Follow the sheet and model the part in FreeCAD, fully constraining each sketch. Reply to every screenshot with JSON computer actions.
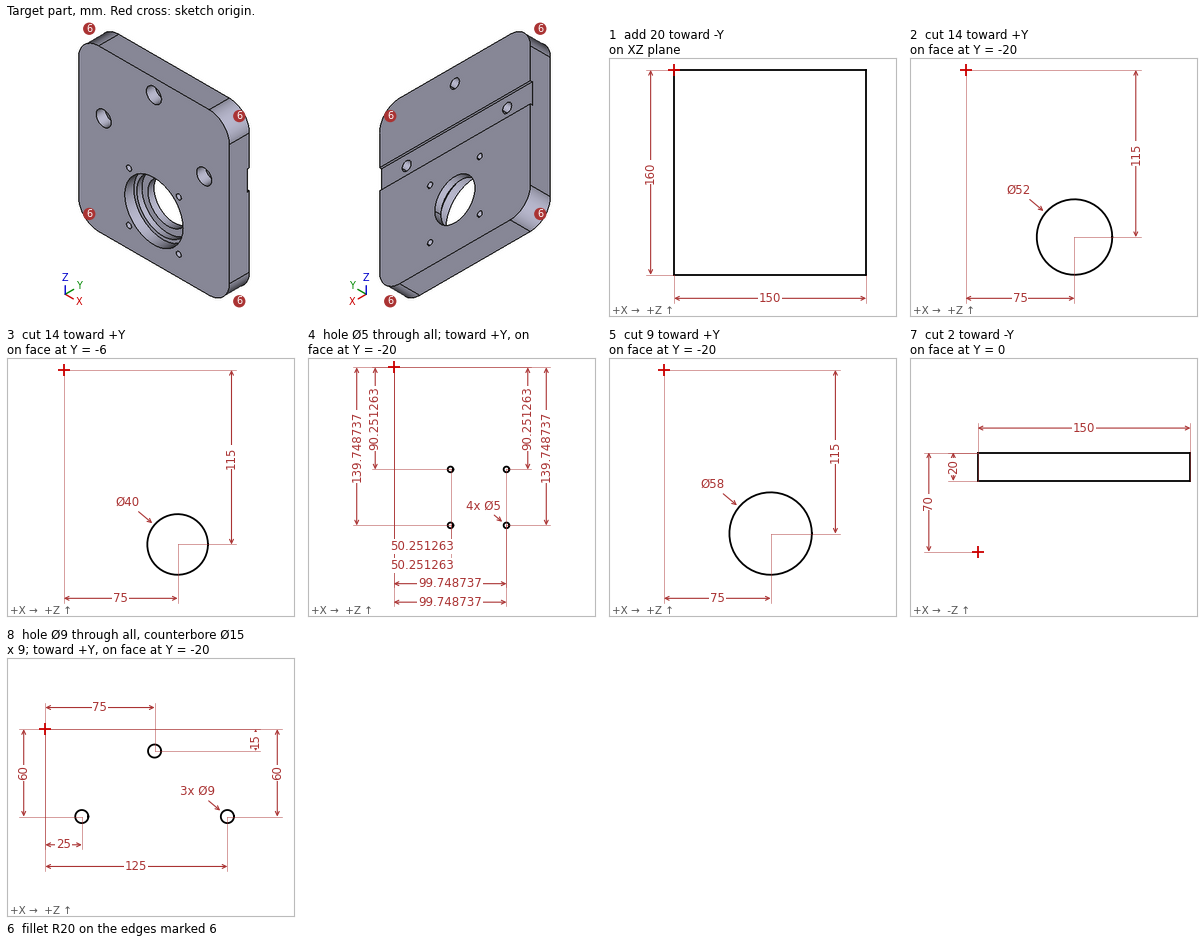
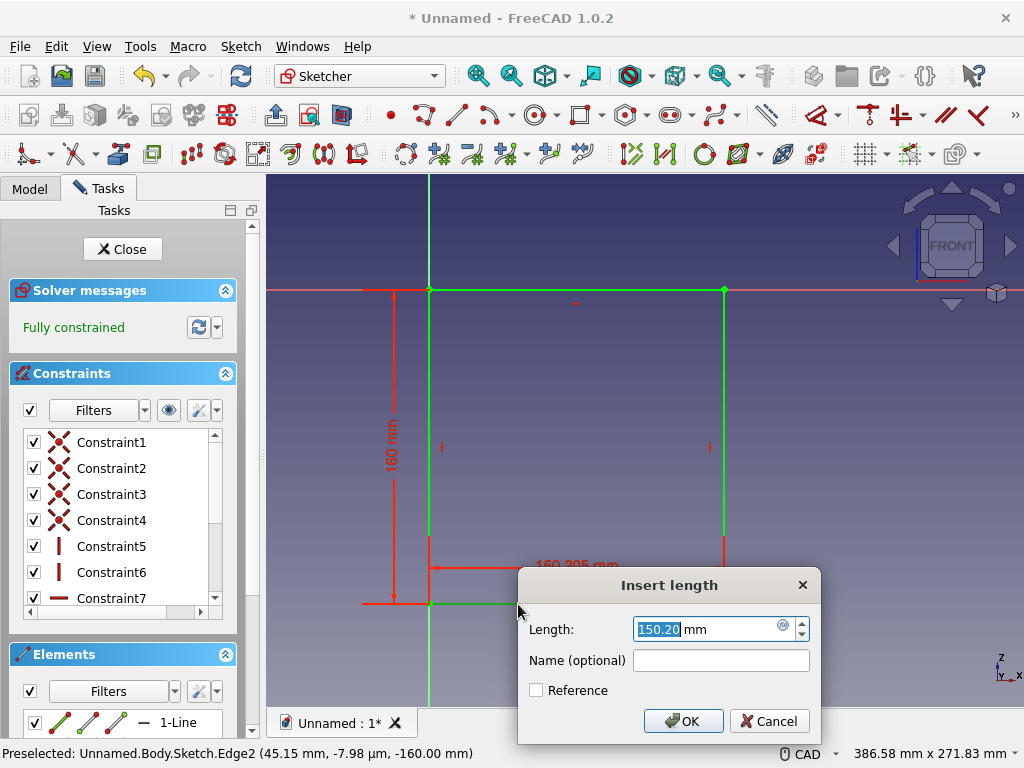
{"action": "type", "text": "150"}
{"action": "key", "text": "Return"}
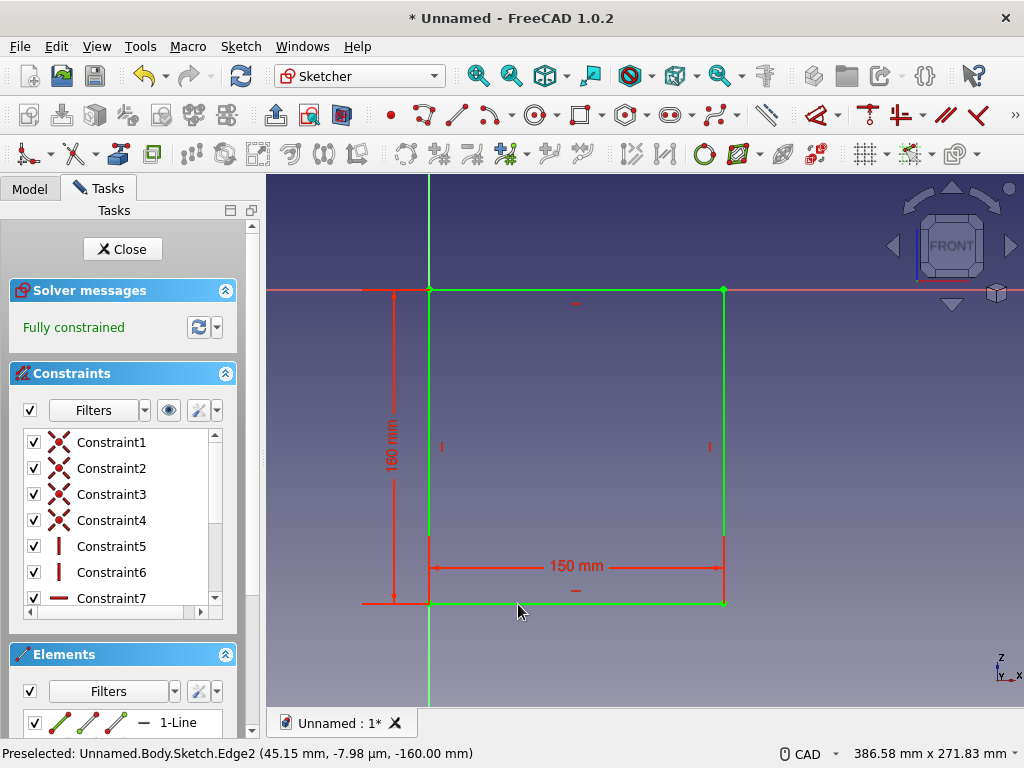
{"action": "left_click", "coordinate": [123, 249]}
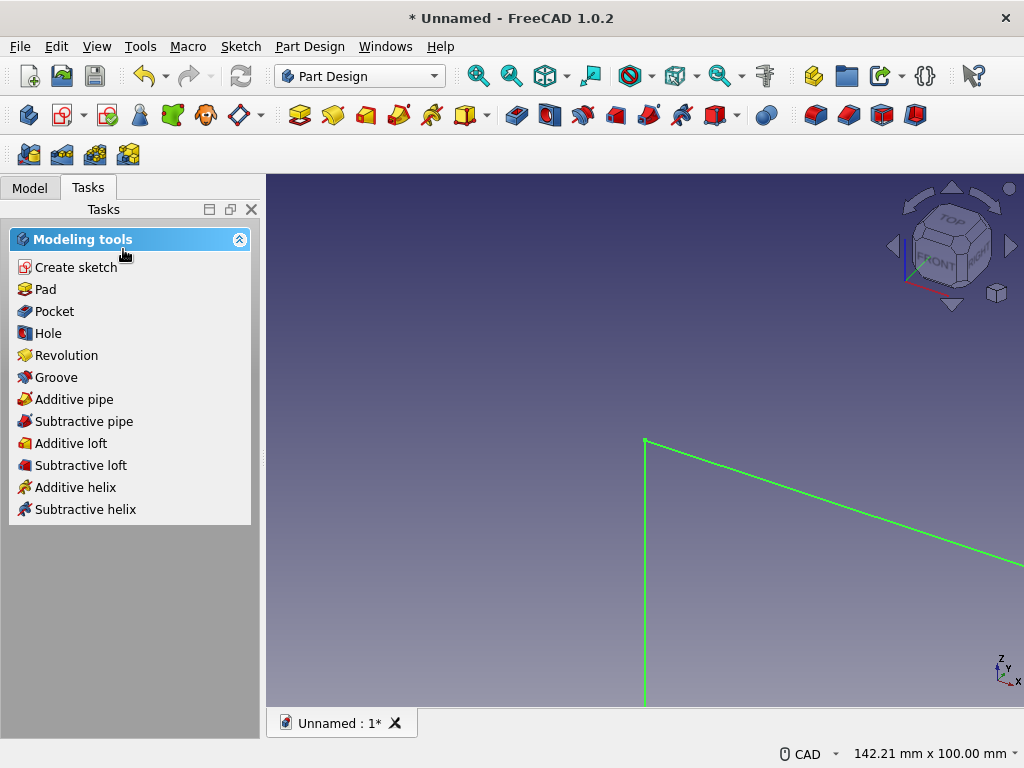
{"action": "left_click", "coordinate": [300, 116]}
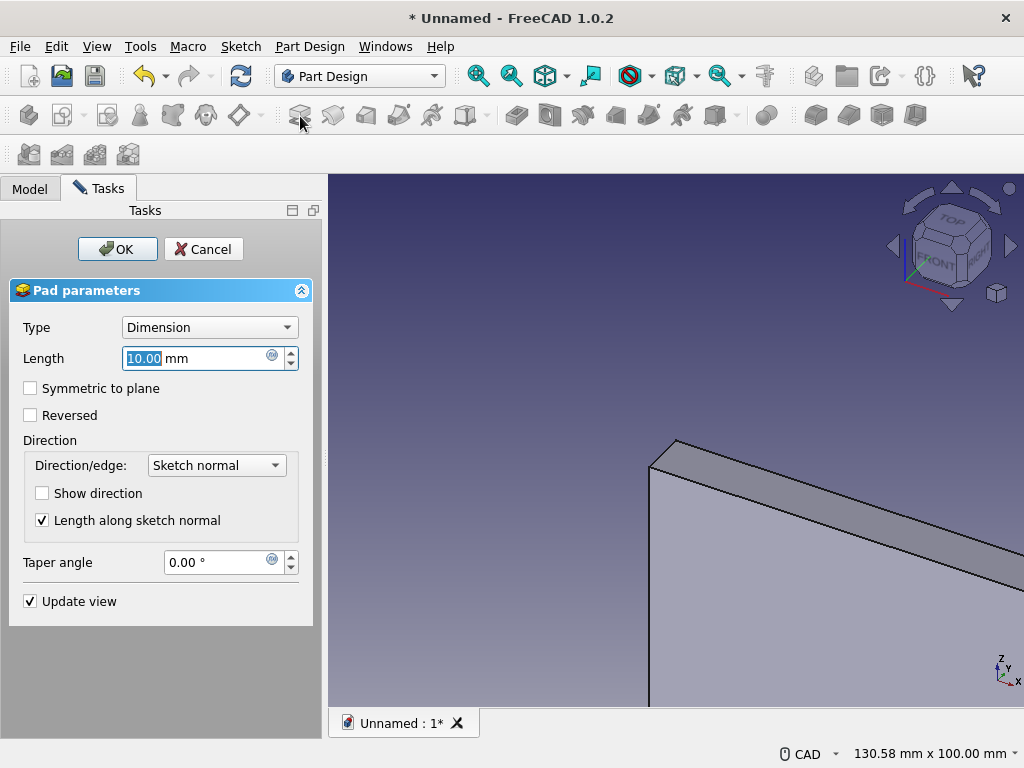
{"action": "type", "text": "20"}
{"action": "key", "text": "Tab"}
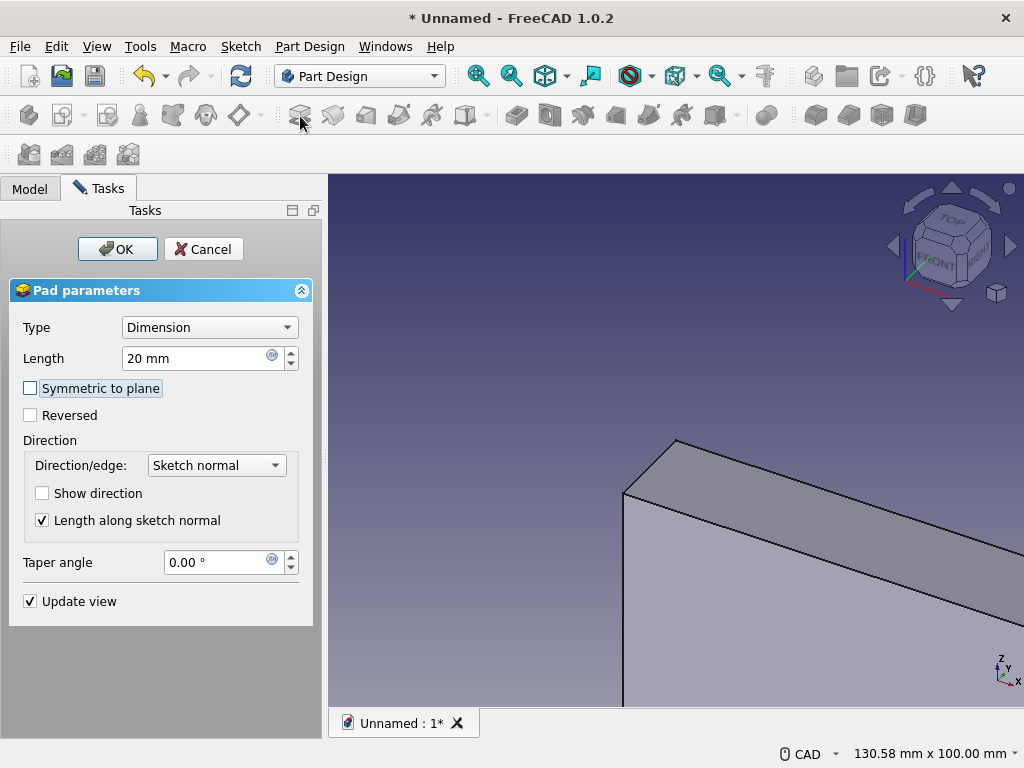
{"action": "left_click", "coordinate": [118, 249]}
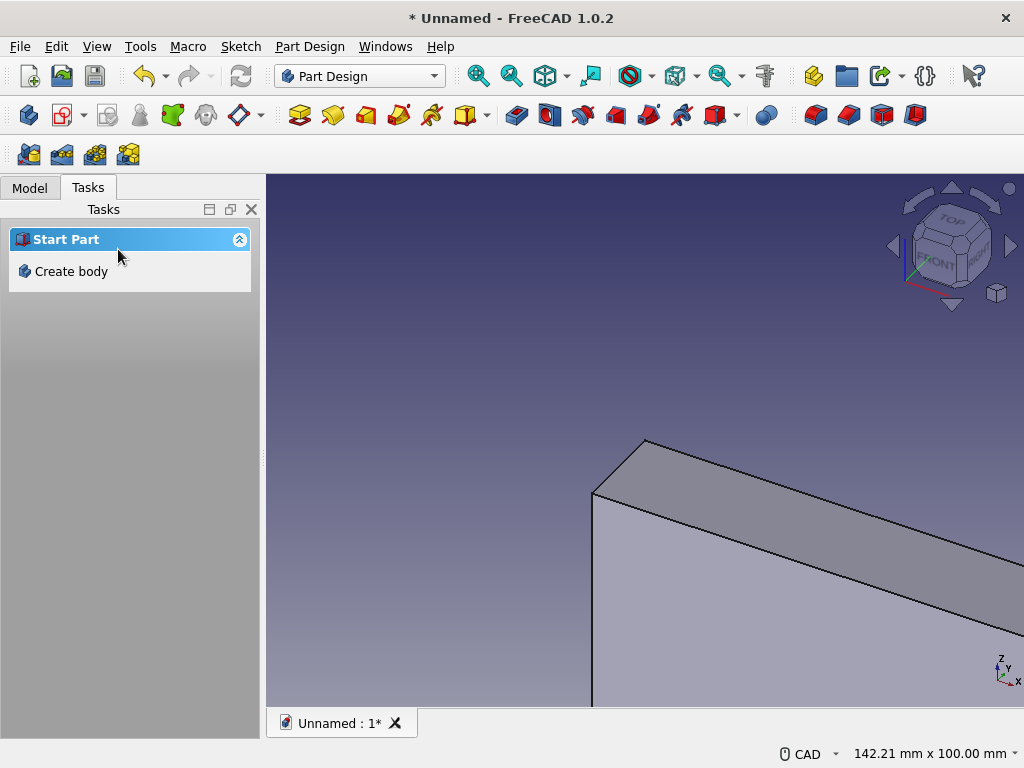
{"action": "left_click", "coordinate": [479, 76]}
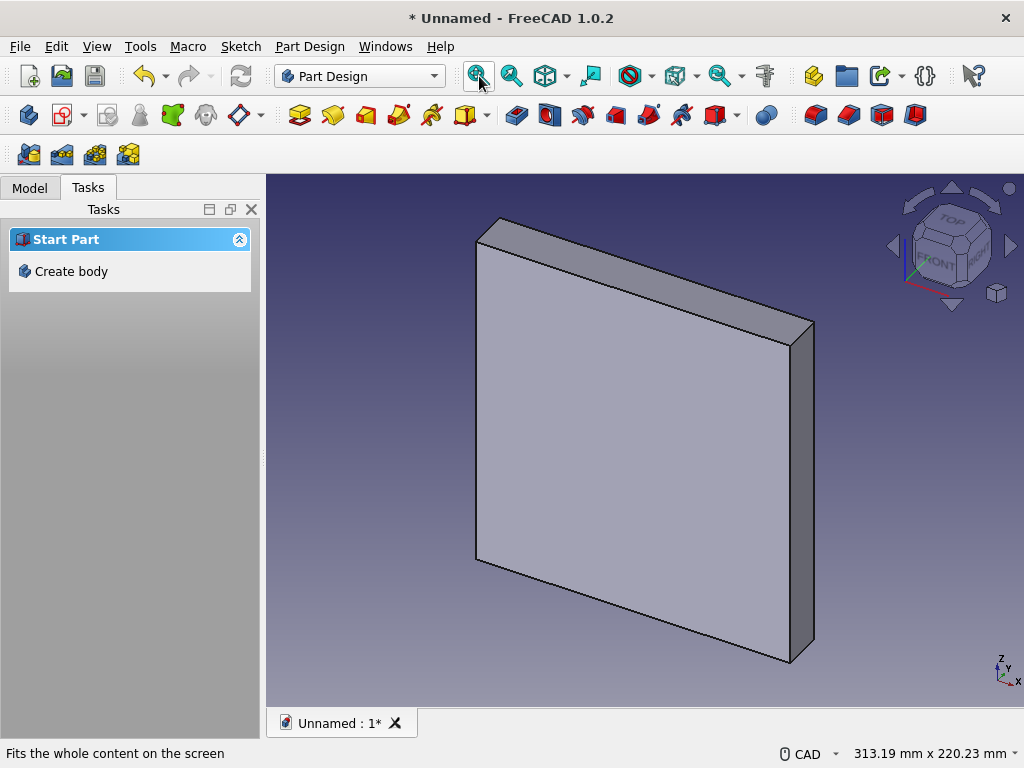
{"action": "left_click", "coordinate": [633, 452]}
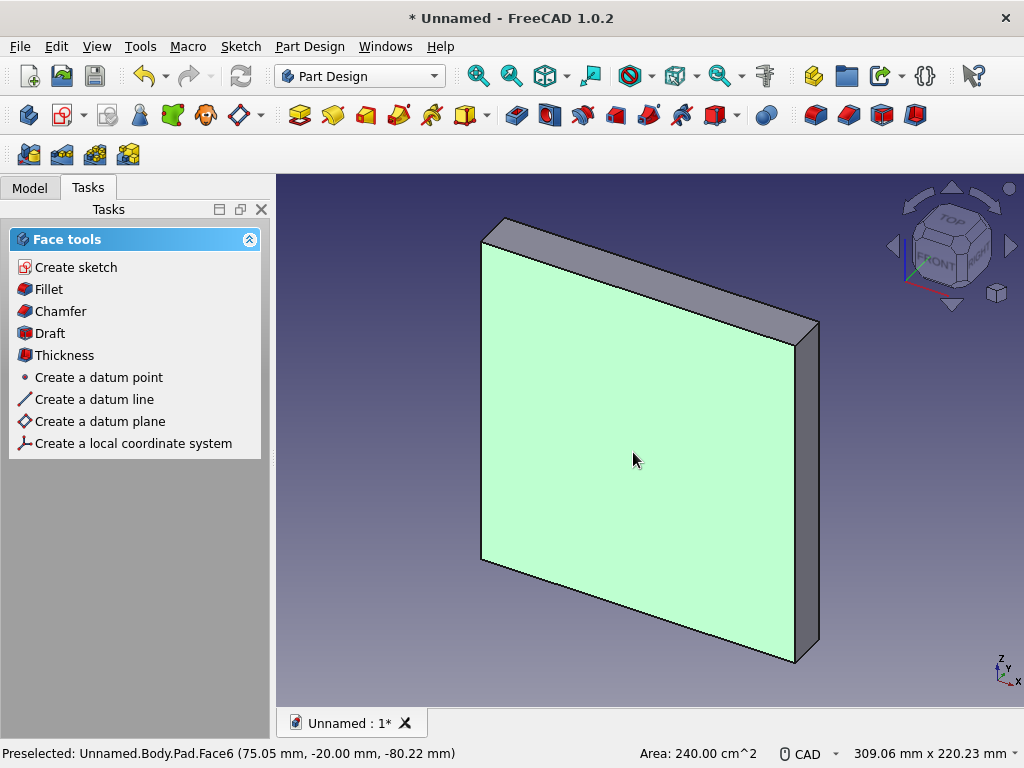
{"action": "left_click", "coordinate": [62, 116]}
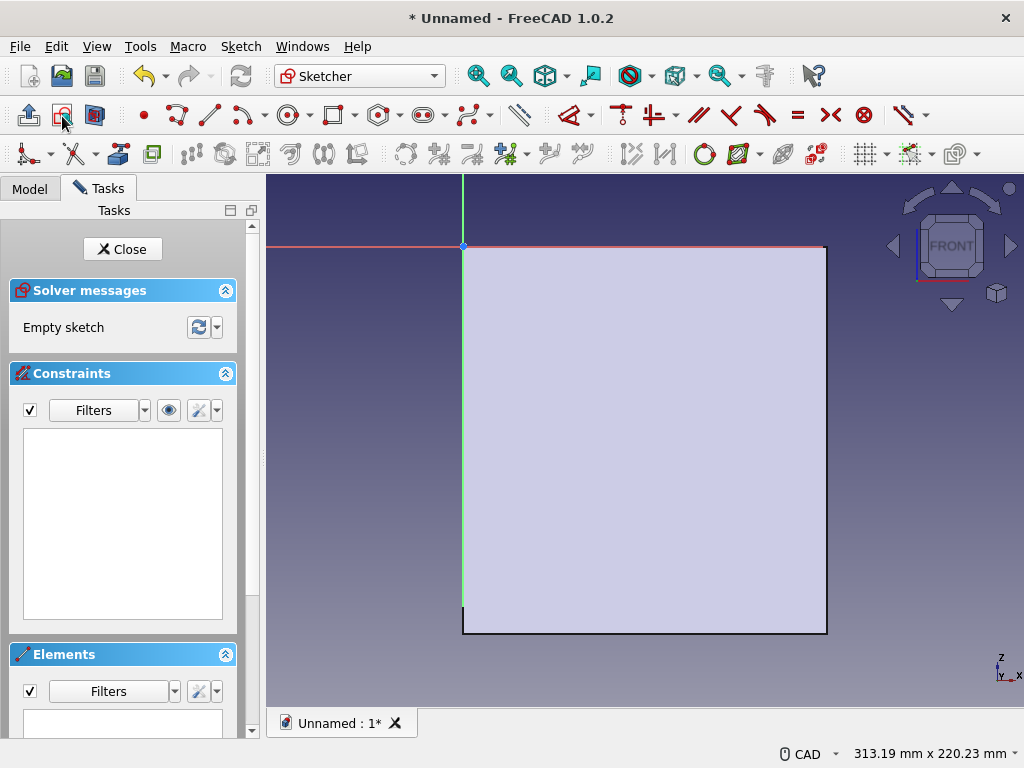
{"action": "scroll", "coordinate": [685, 575], "scroll_direction": "up", "scroll_amount": 5}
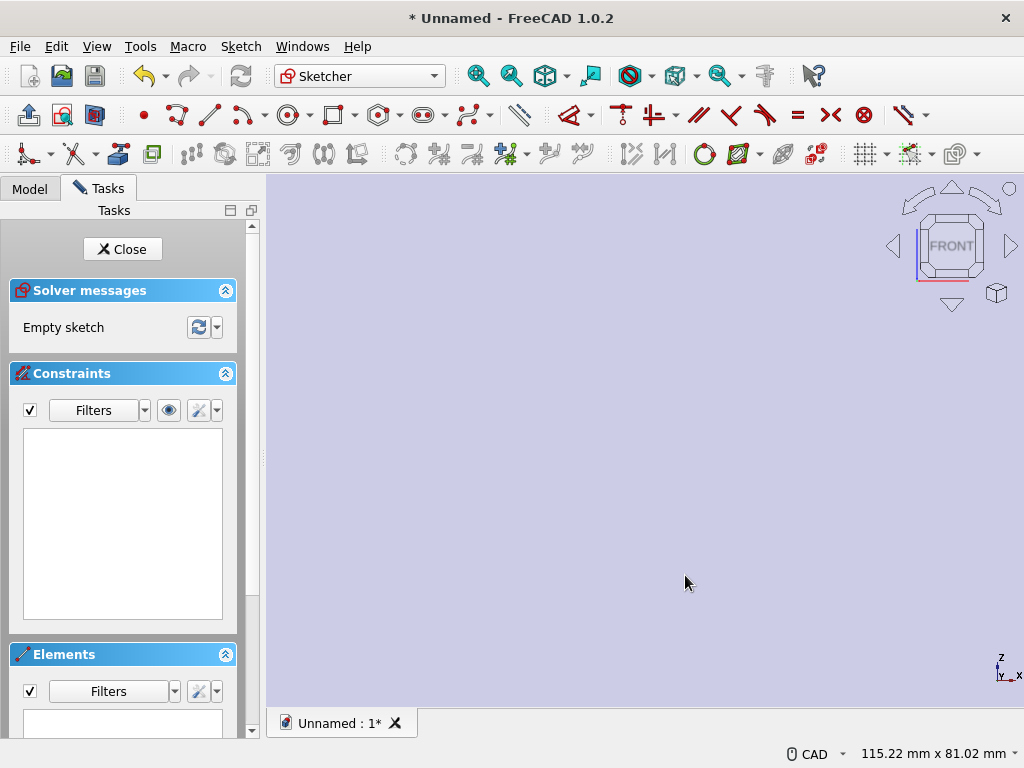
{"action": "left_click", "coordinate": [288, 116]}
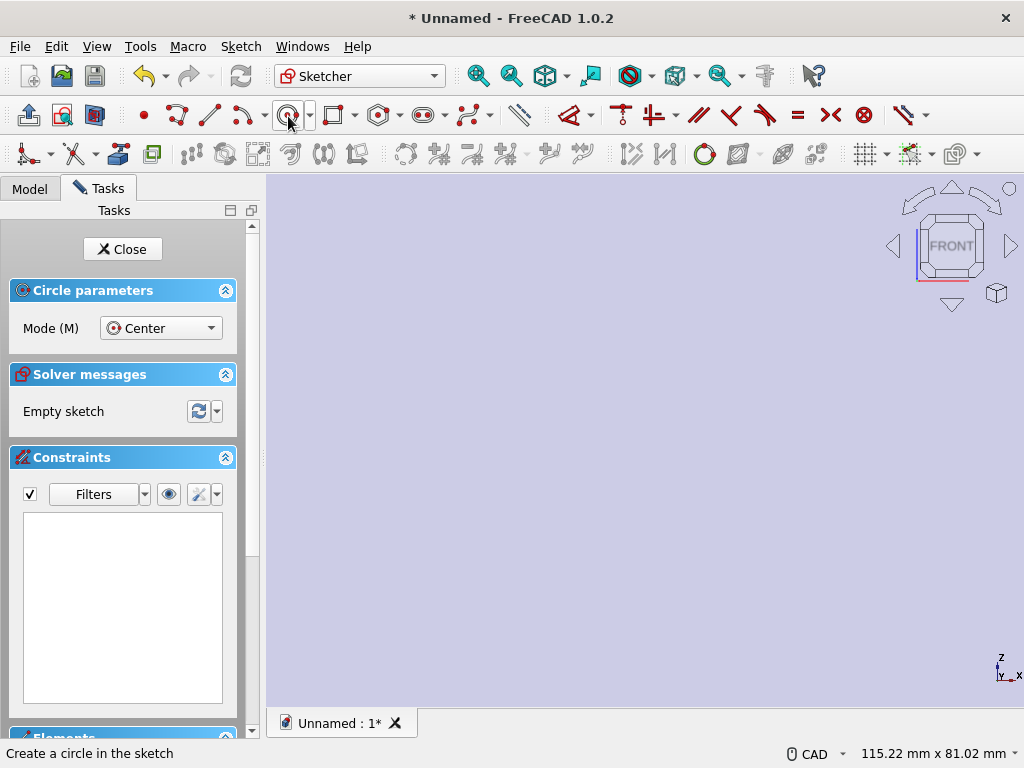
{"action": "left_click", "coordinate": [575, 438]}
{"action": "left_click", "coordinate": [696, 317]}
{"action": "key", "text": "Escape"}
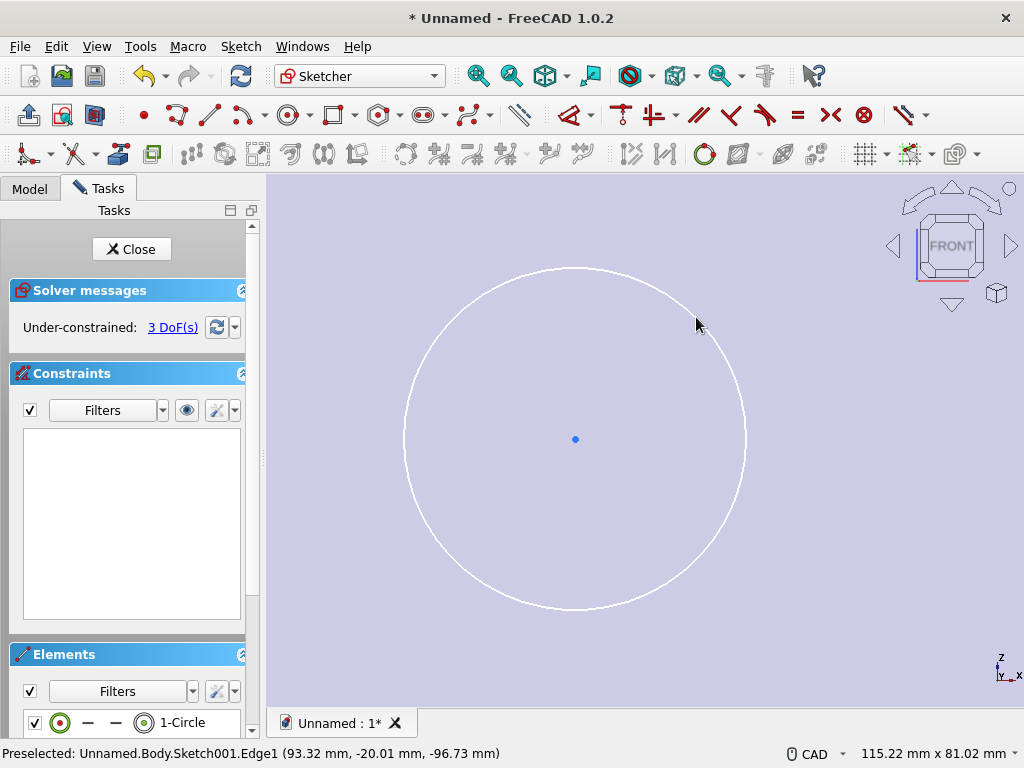
{"action": "left_click", "coordinate": [696, 318]}